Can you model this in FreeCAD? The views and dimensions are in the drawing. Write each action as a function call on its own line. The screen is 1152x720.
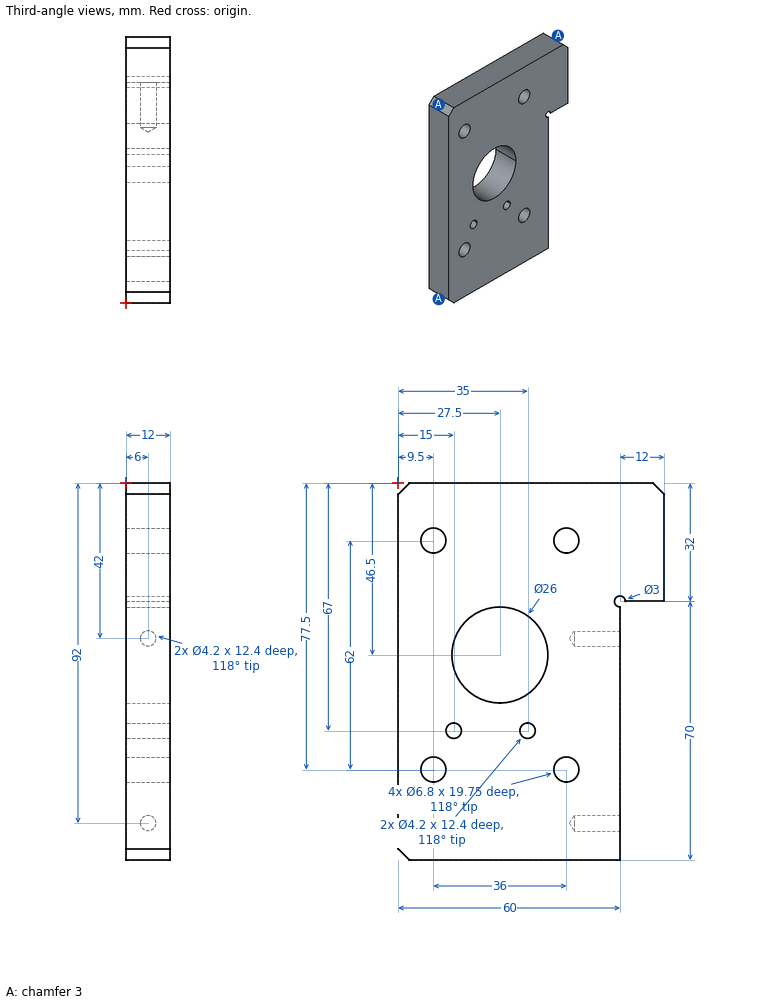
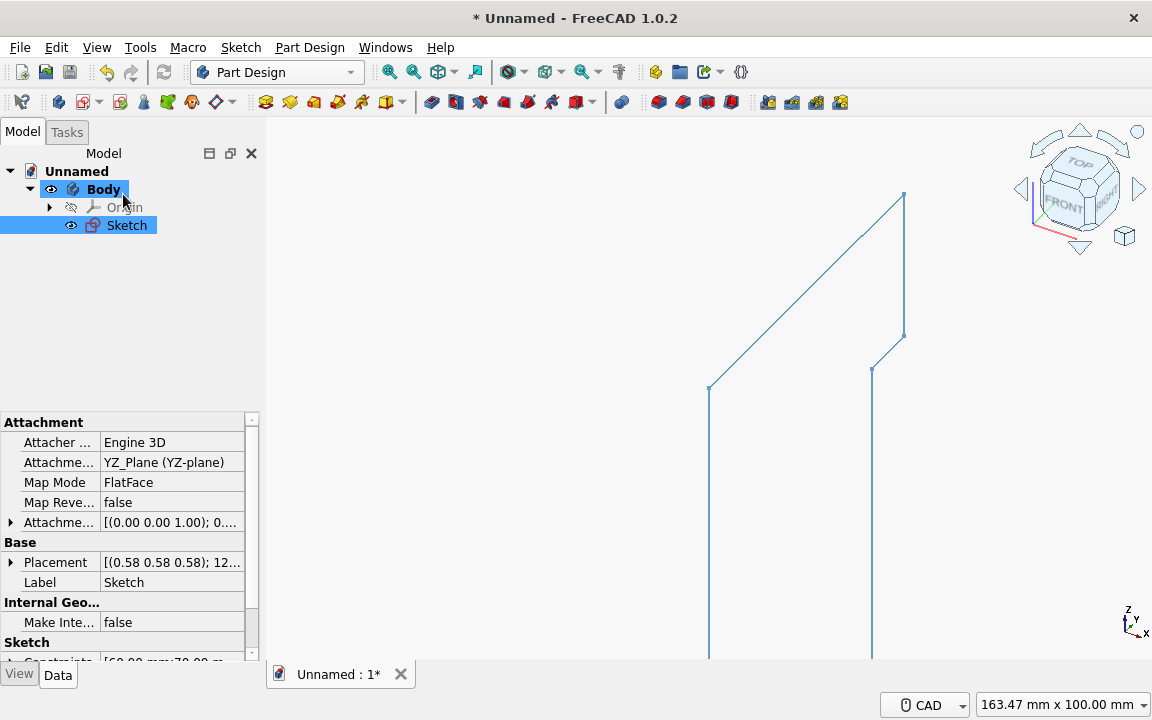
click(266, 102)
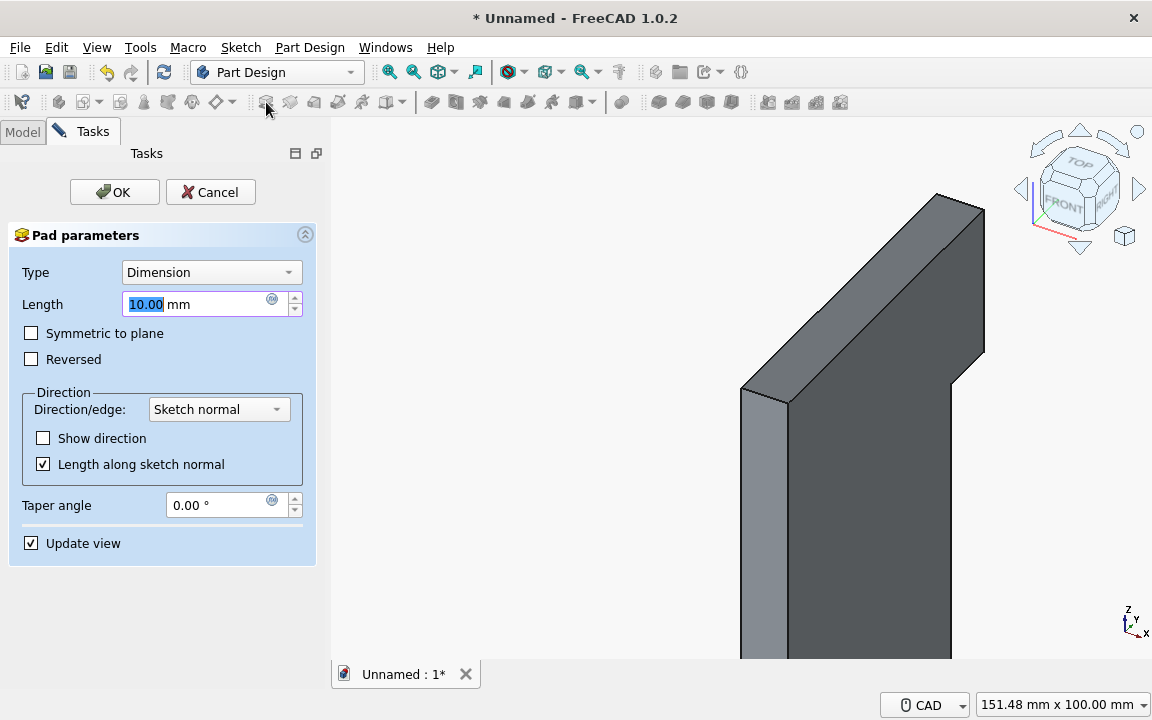
text(12)
key(Tab)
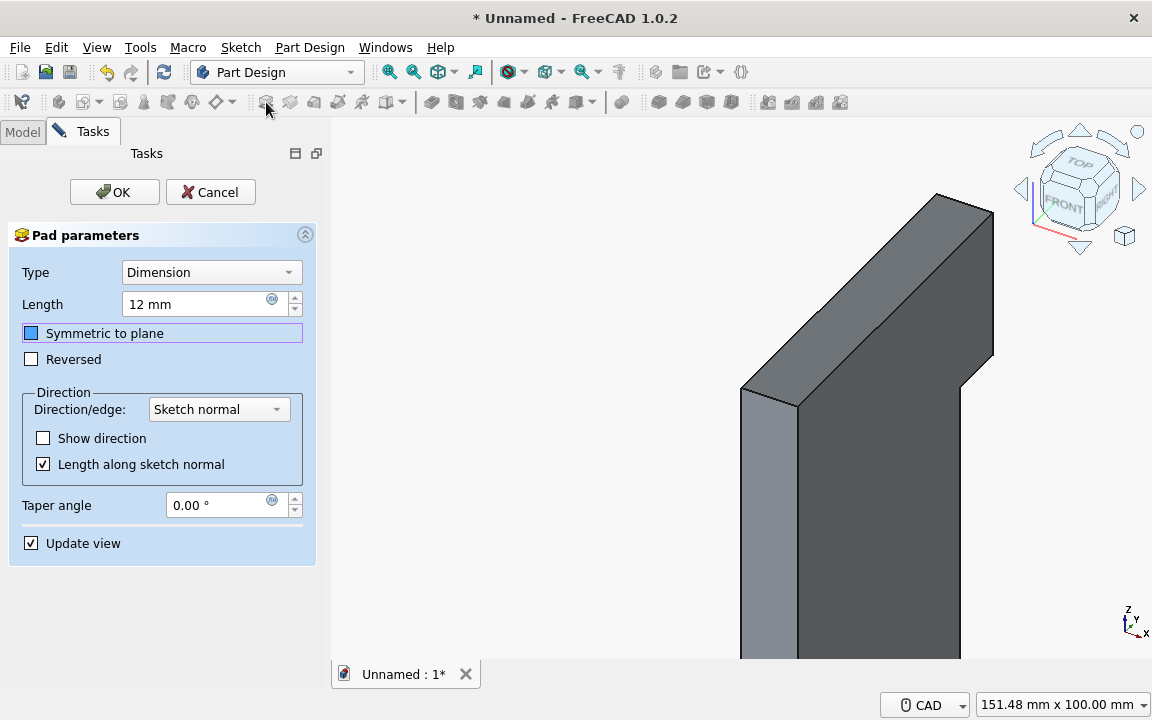
click(115, 192)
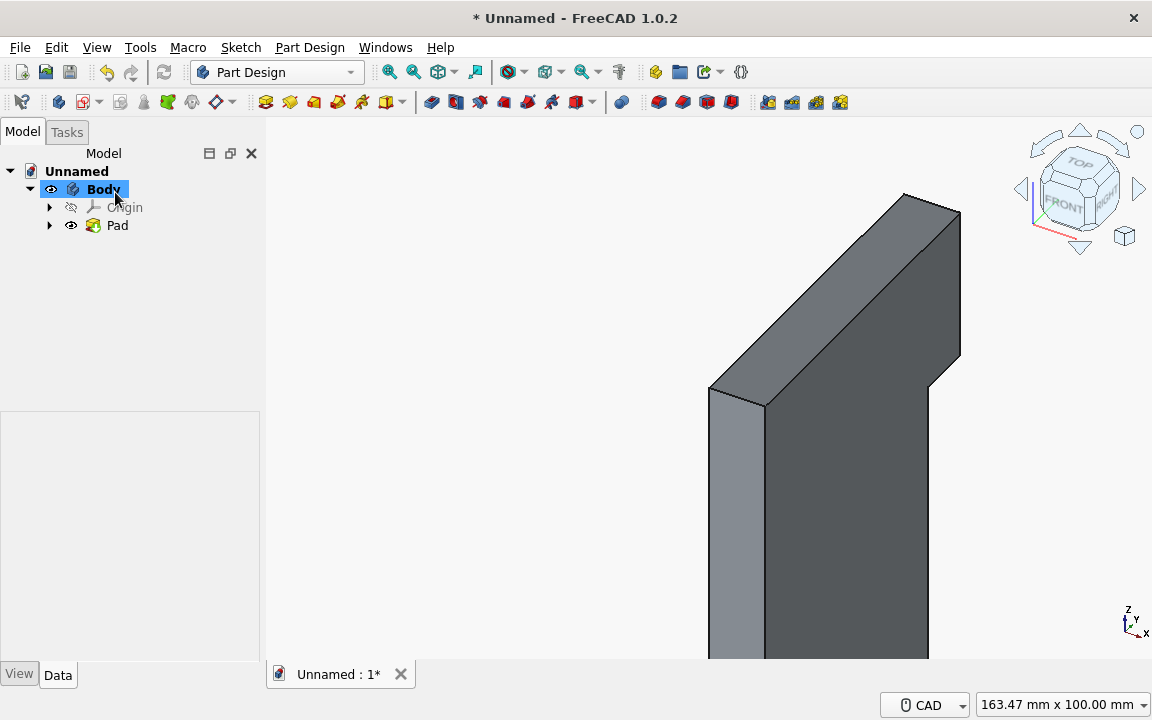
click(390, 72)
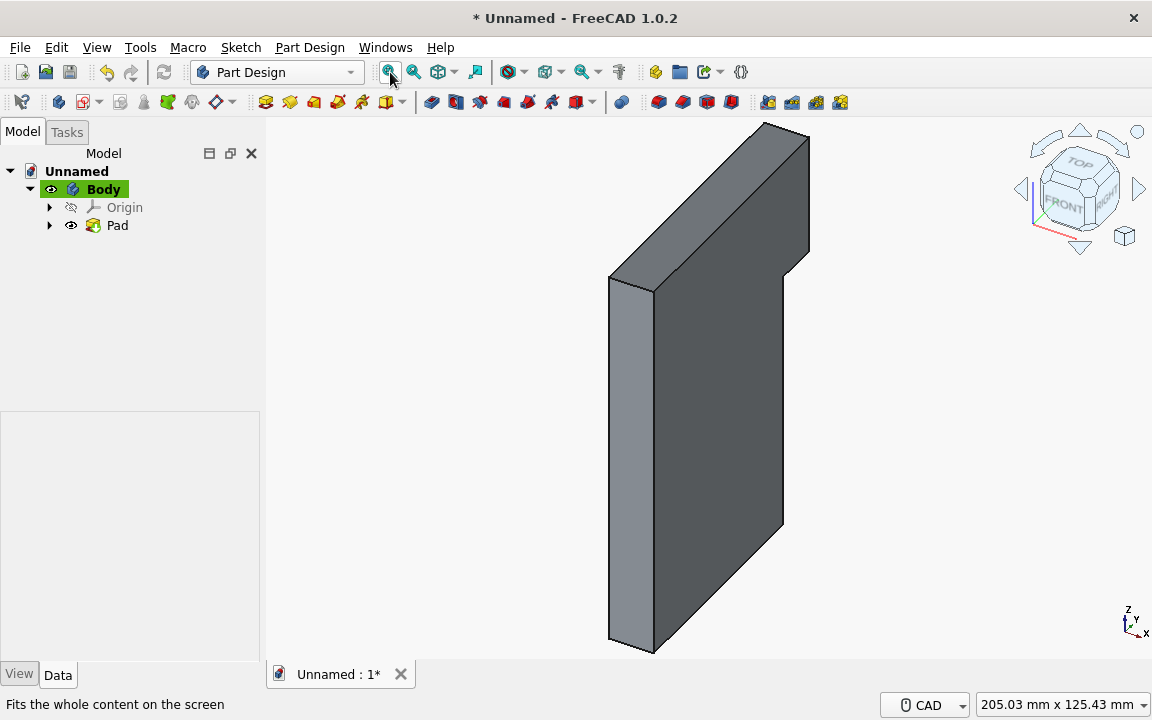
click(709, 468)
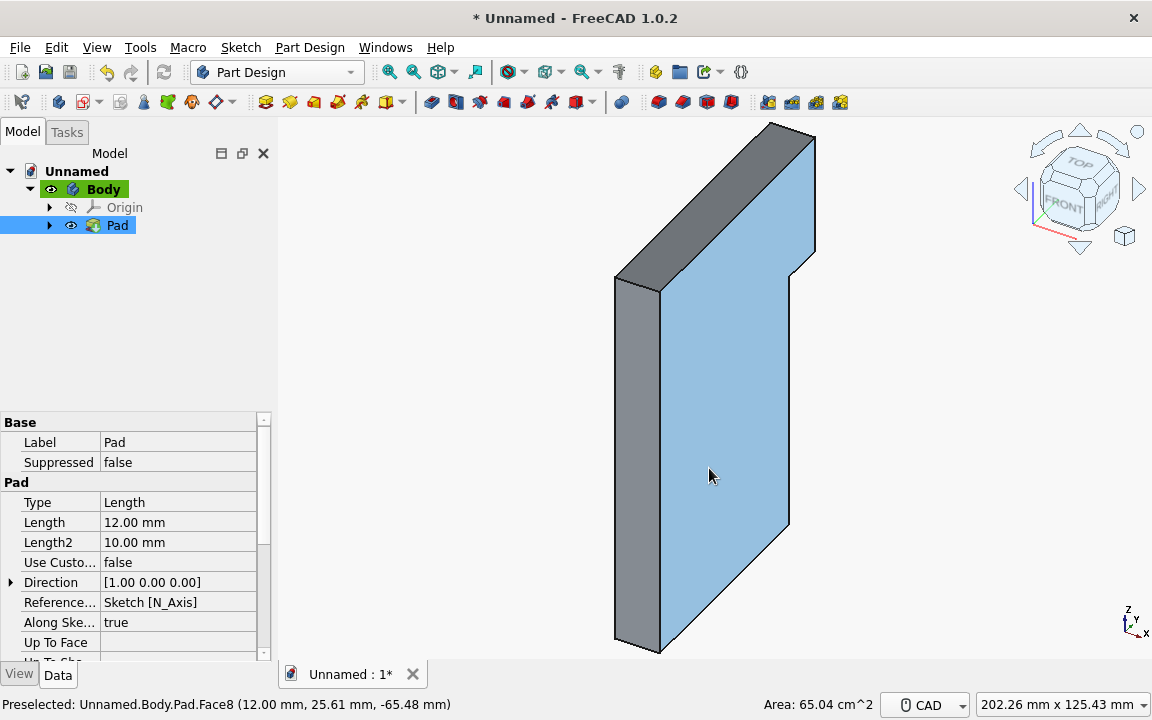
click(84, 102)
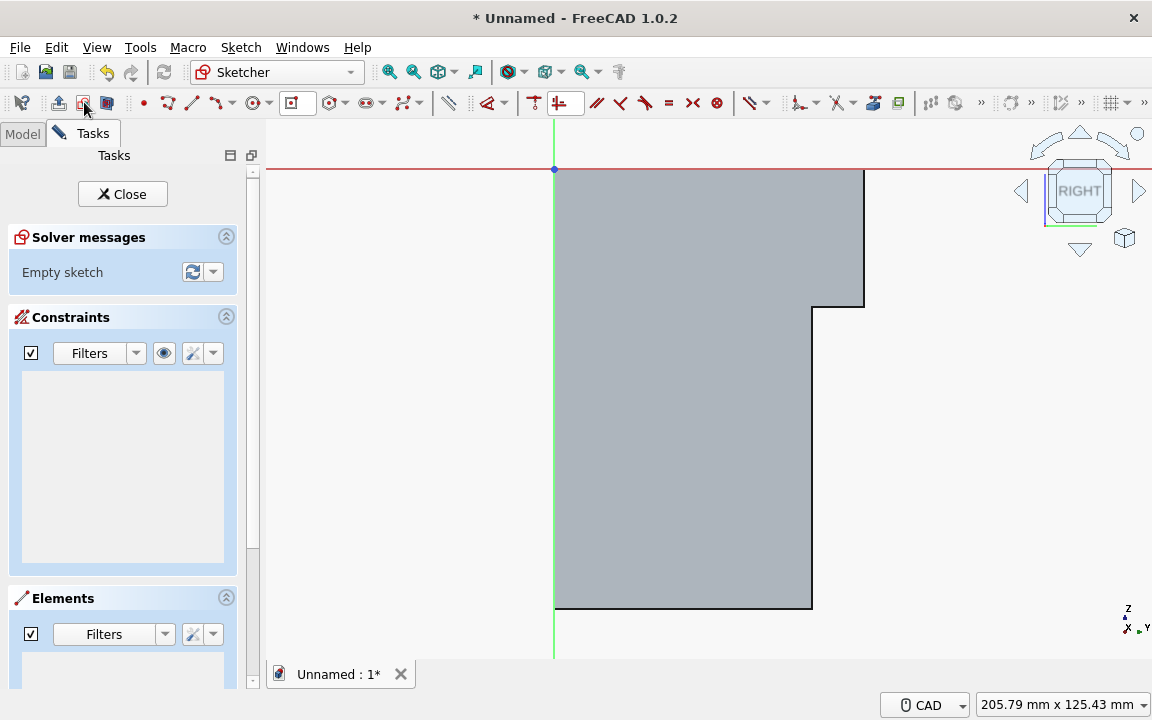
scroll(644, 147, up, 1)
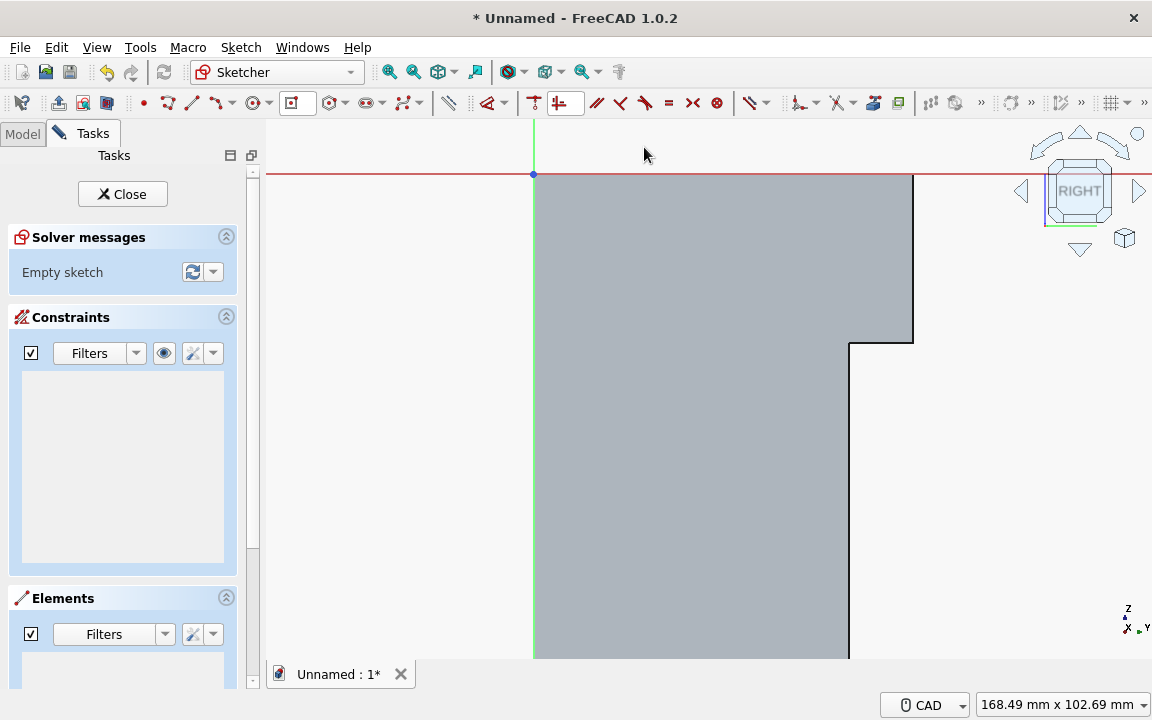
key(g)
key(c)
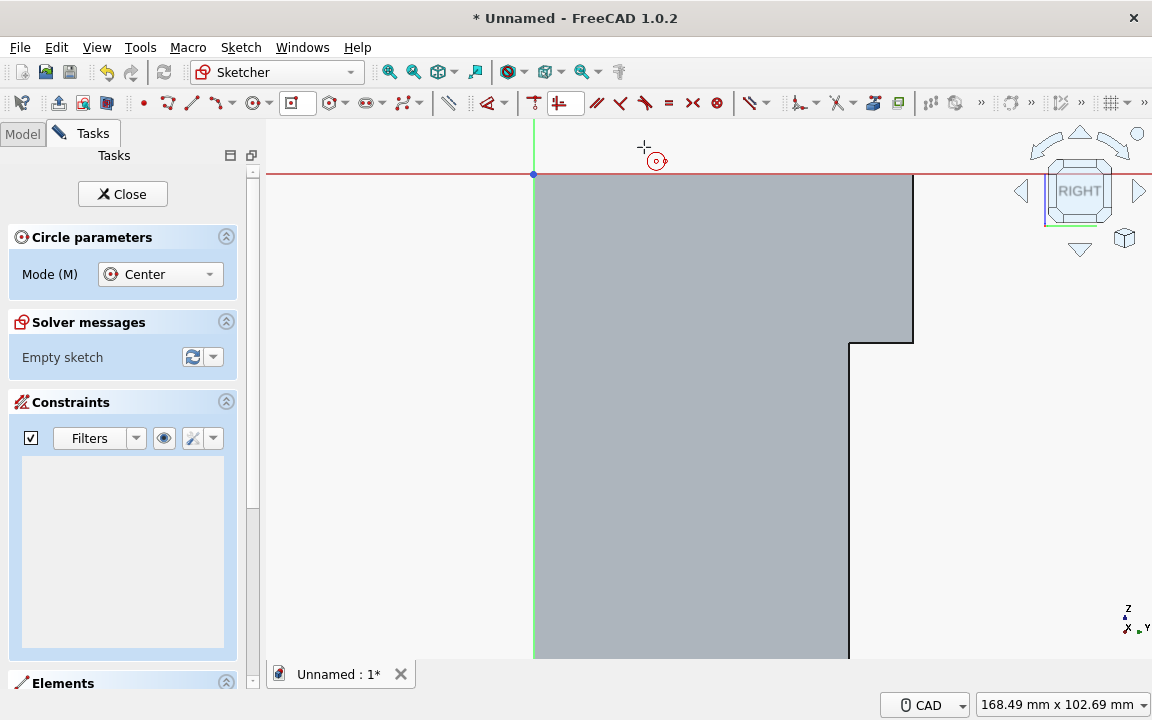
click(679, 419)
move(727, 371)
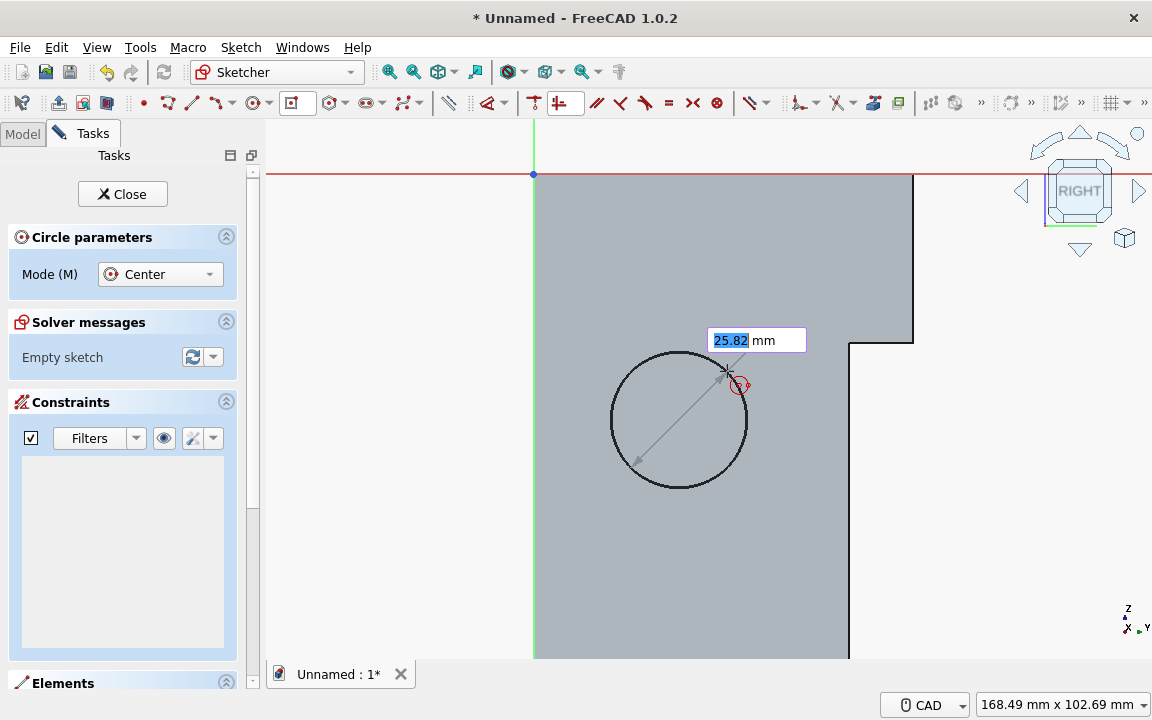
text(26)
key(Return)
key(Escape)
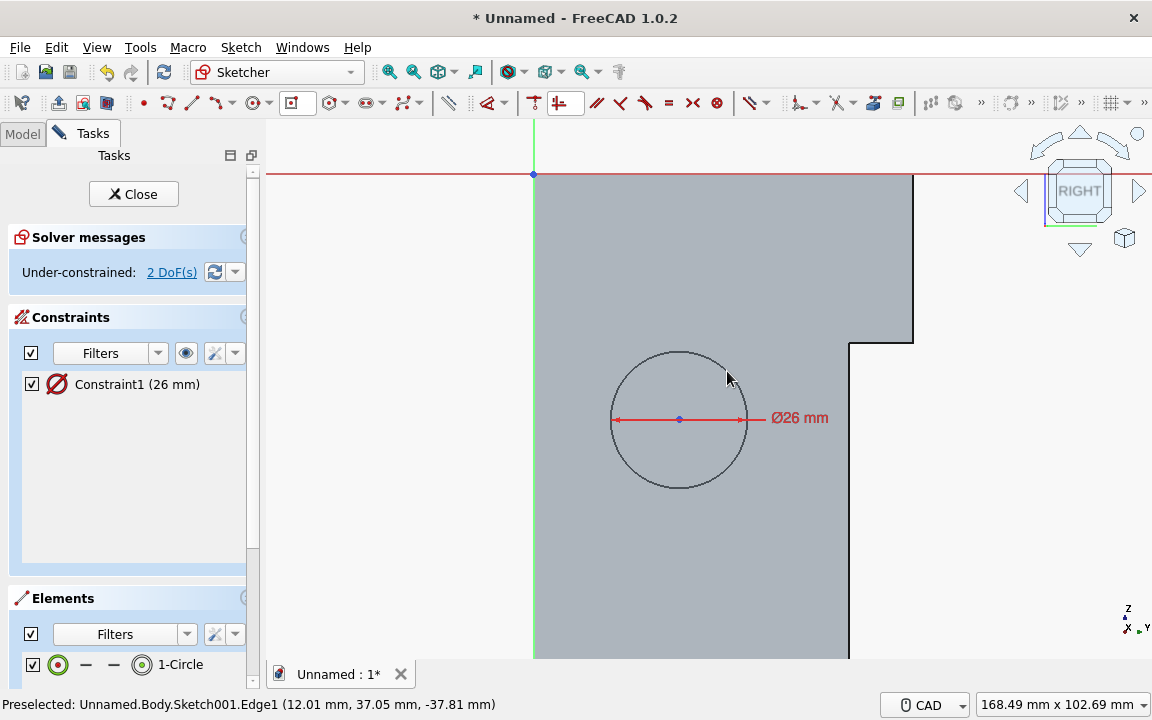
click(679, 420)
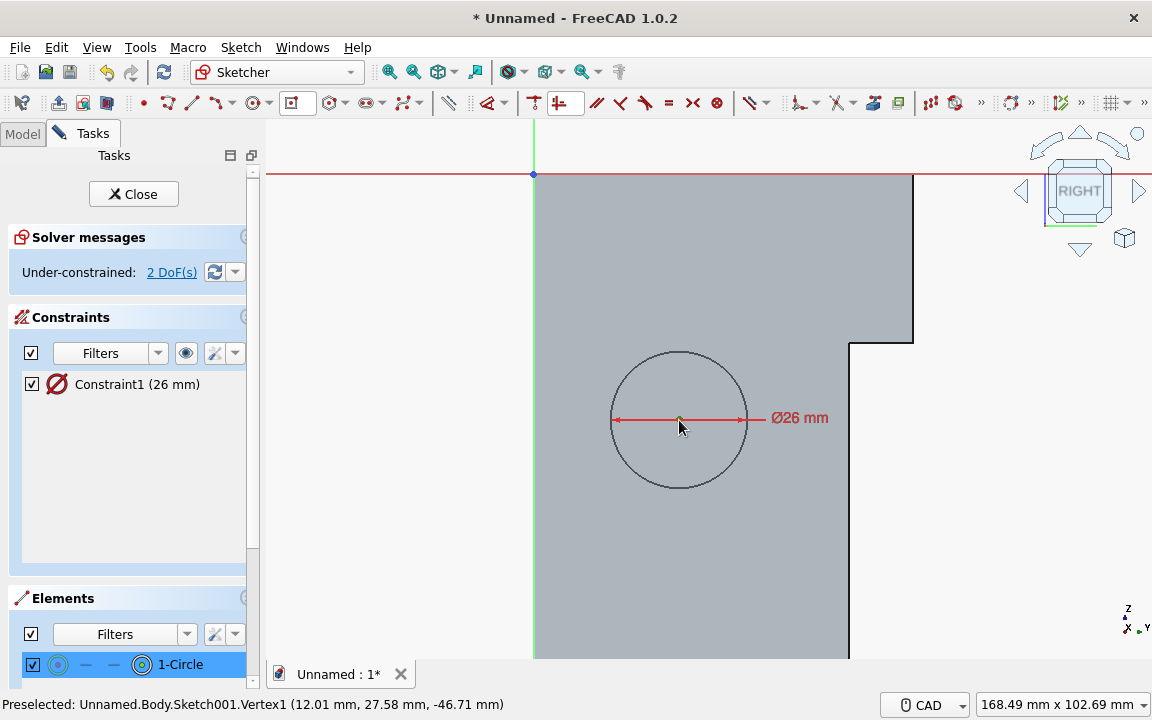
key(l)